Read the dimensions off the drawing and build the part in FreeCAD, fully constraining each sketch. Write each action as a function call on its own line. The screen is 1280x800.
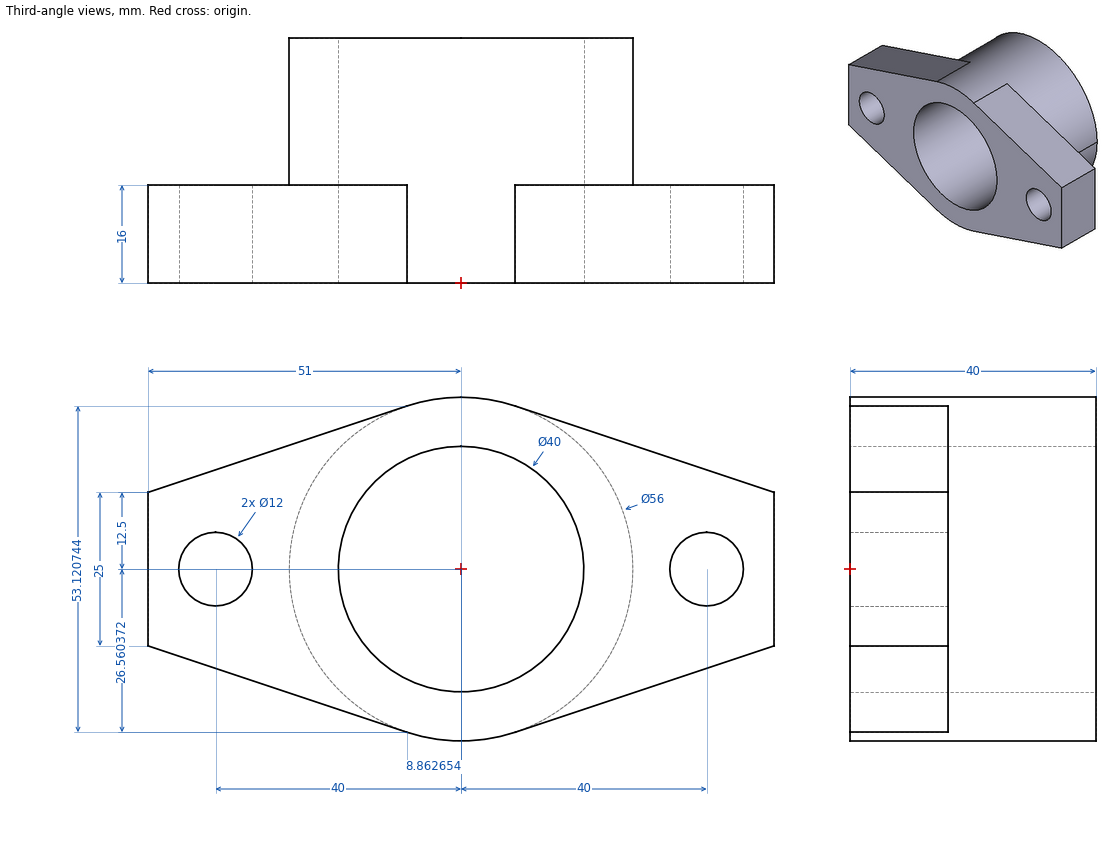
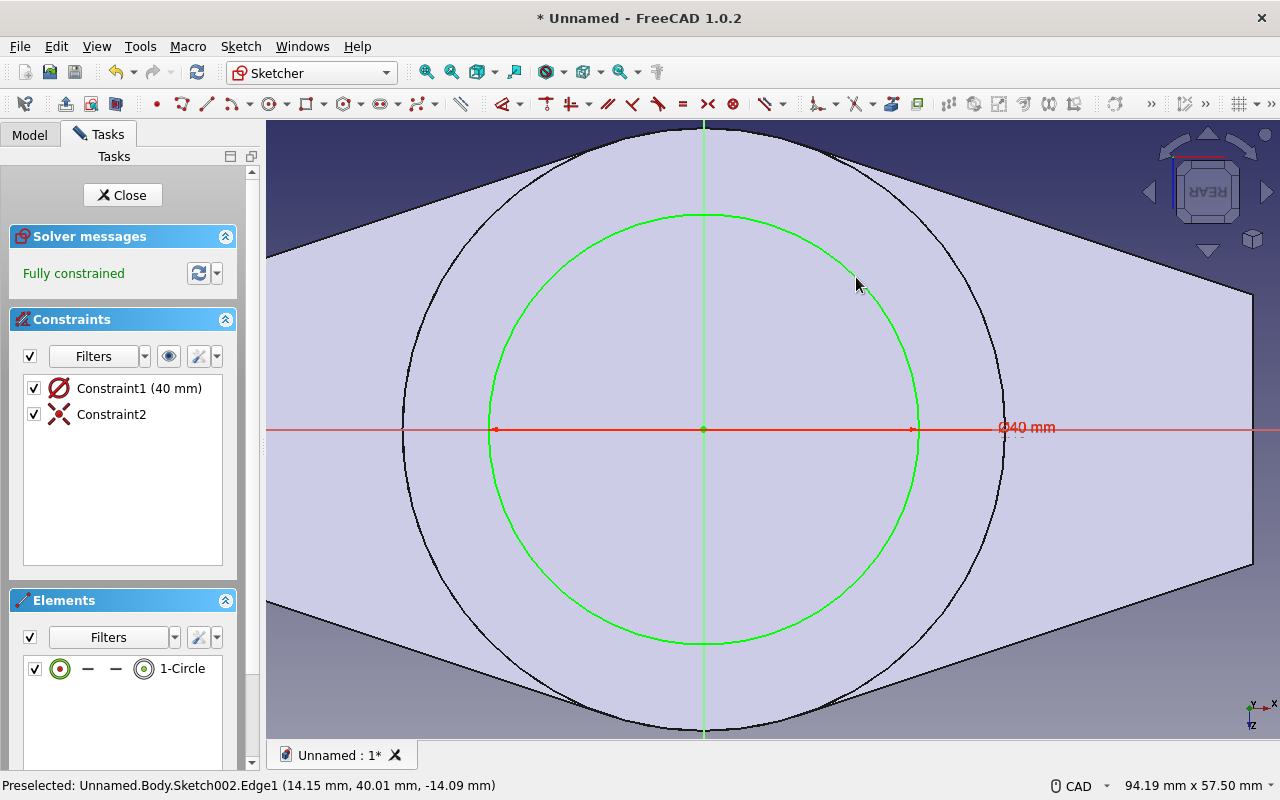
click(123, 195)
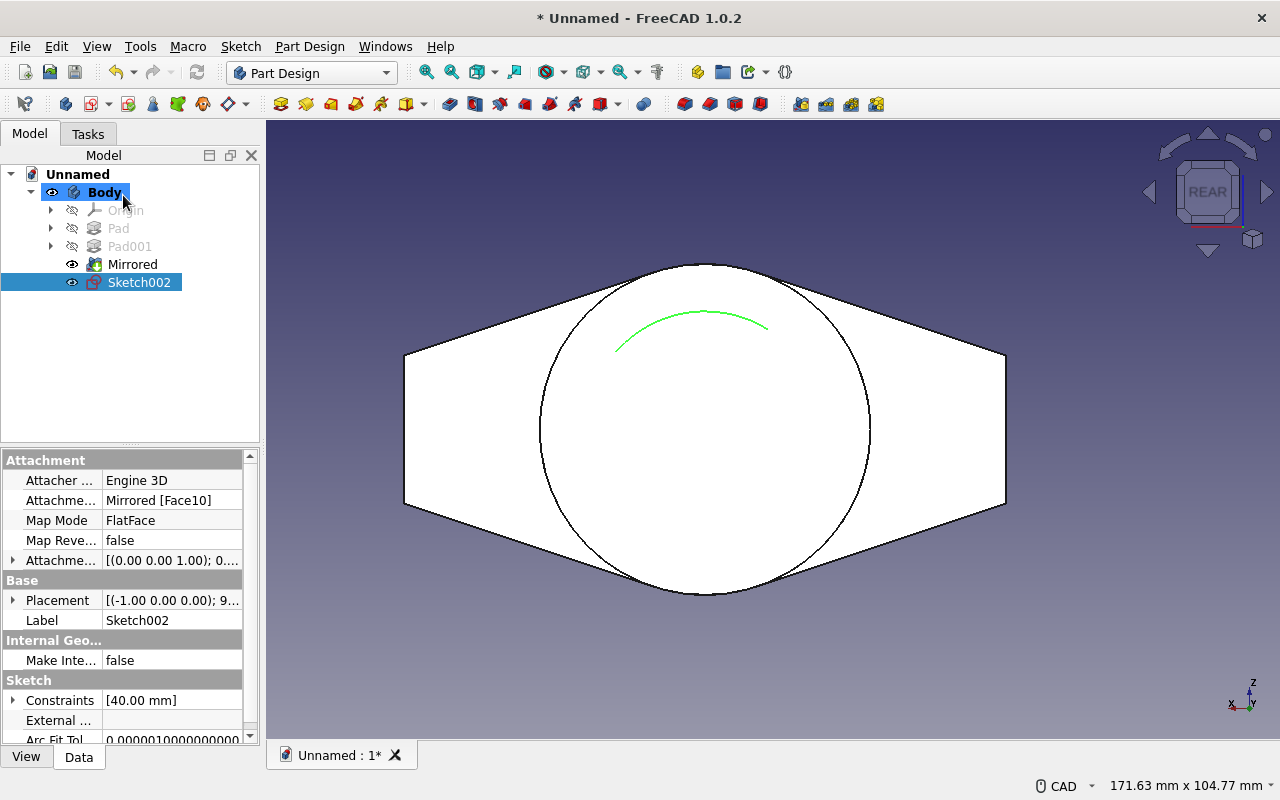
click(450, 104)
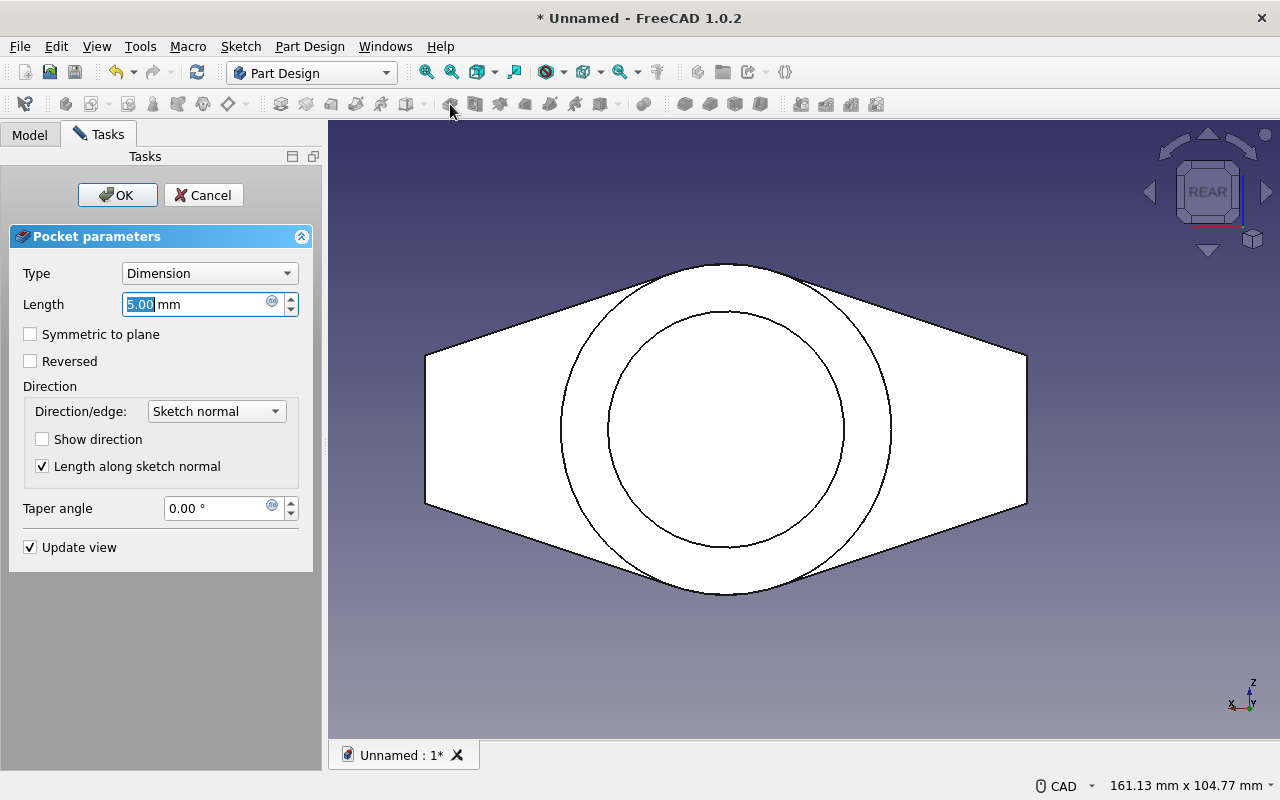
click(210, 274)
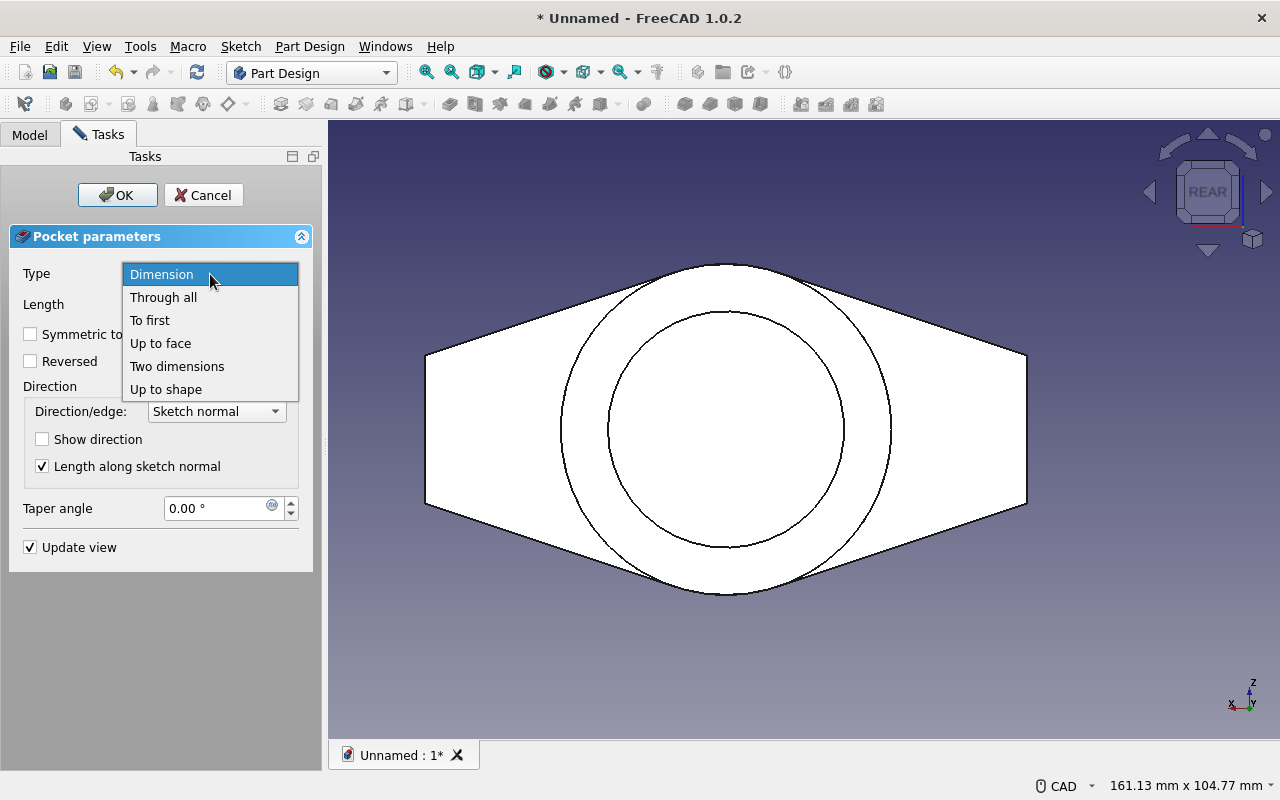
click(208, 298)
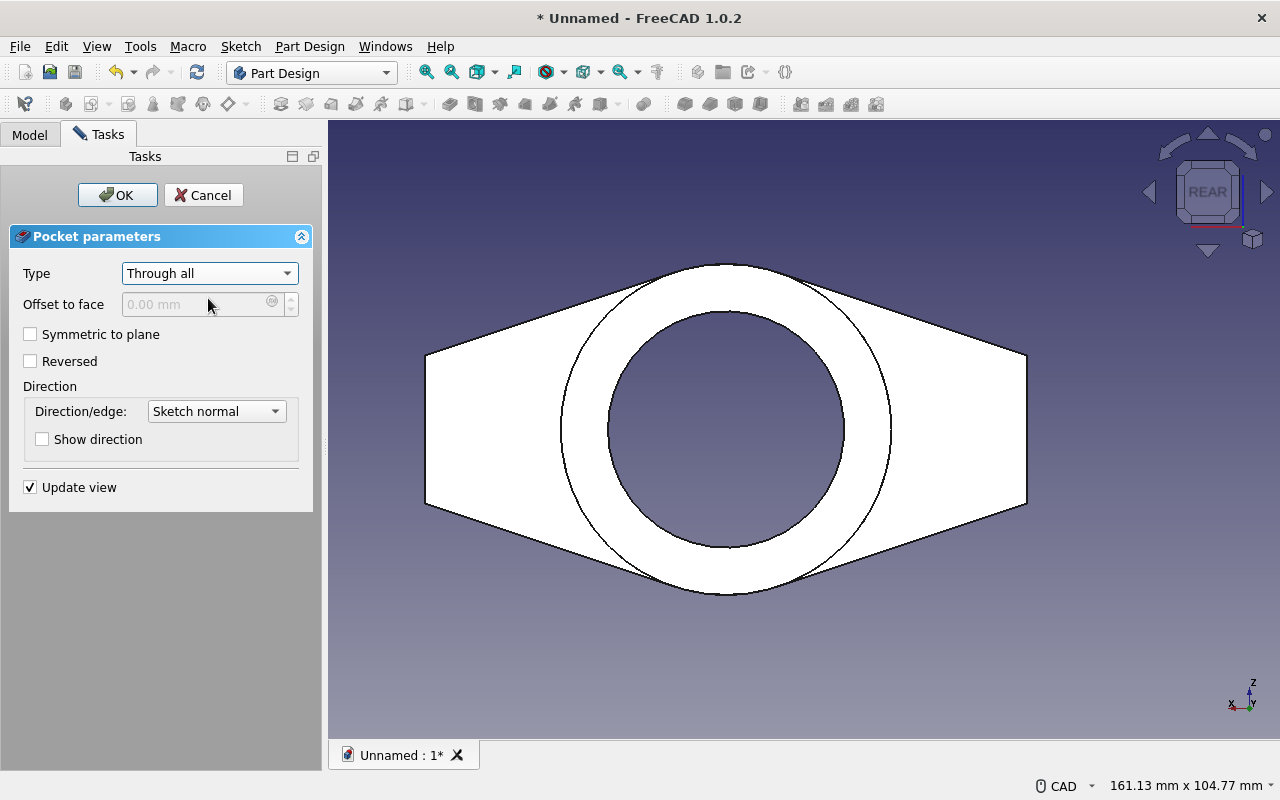
click(118, 195)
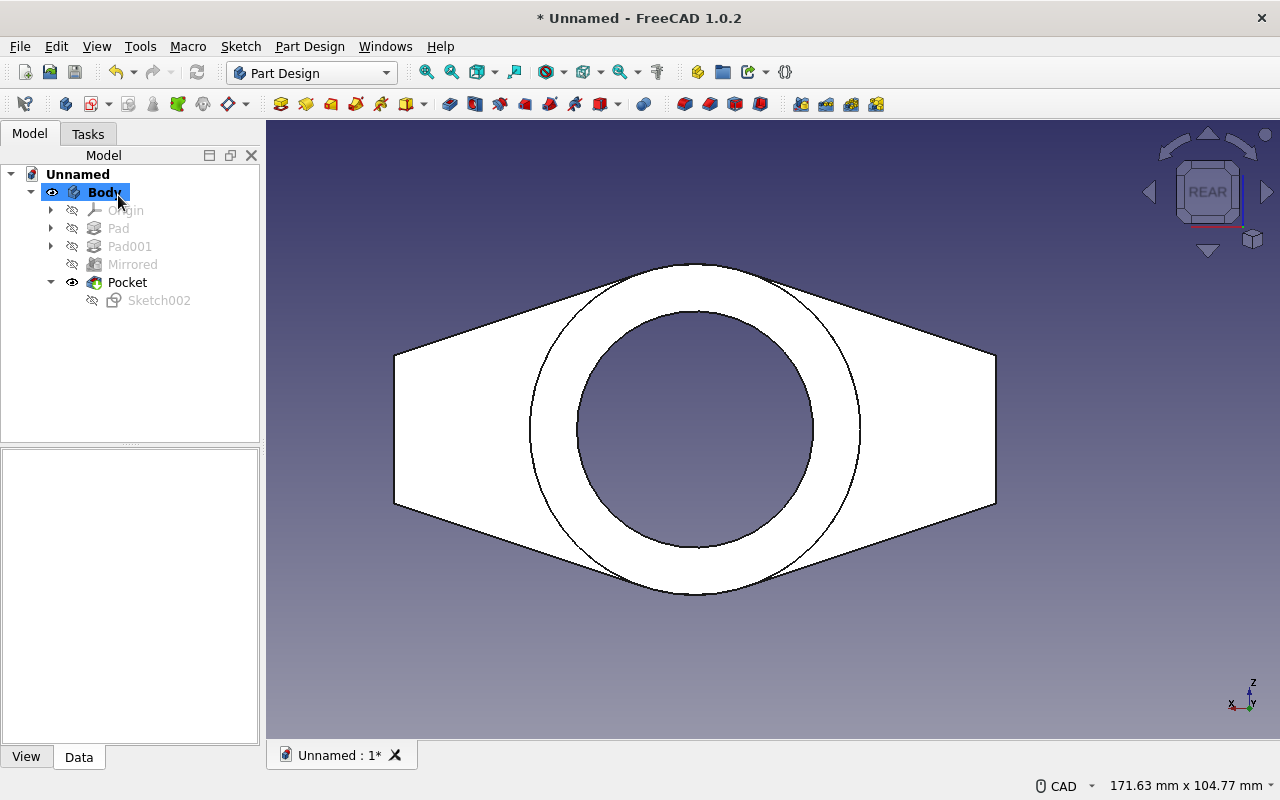
click(447, 429)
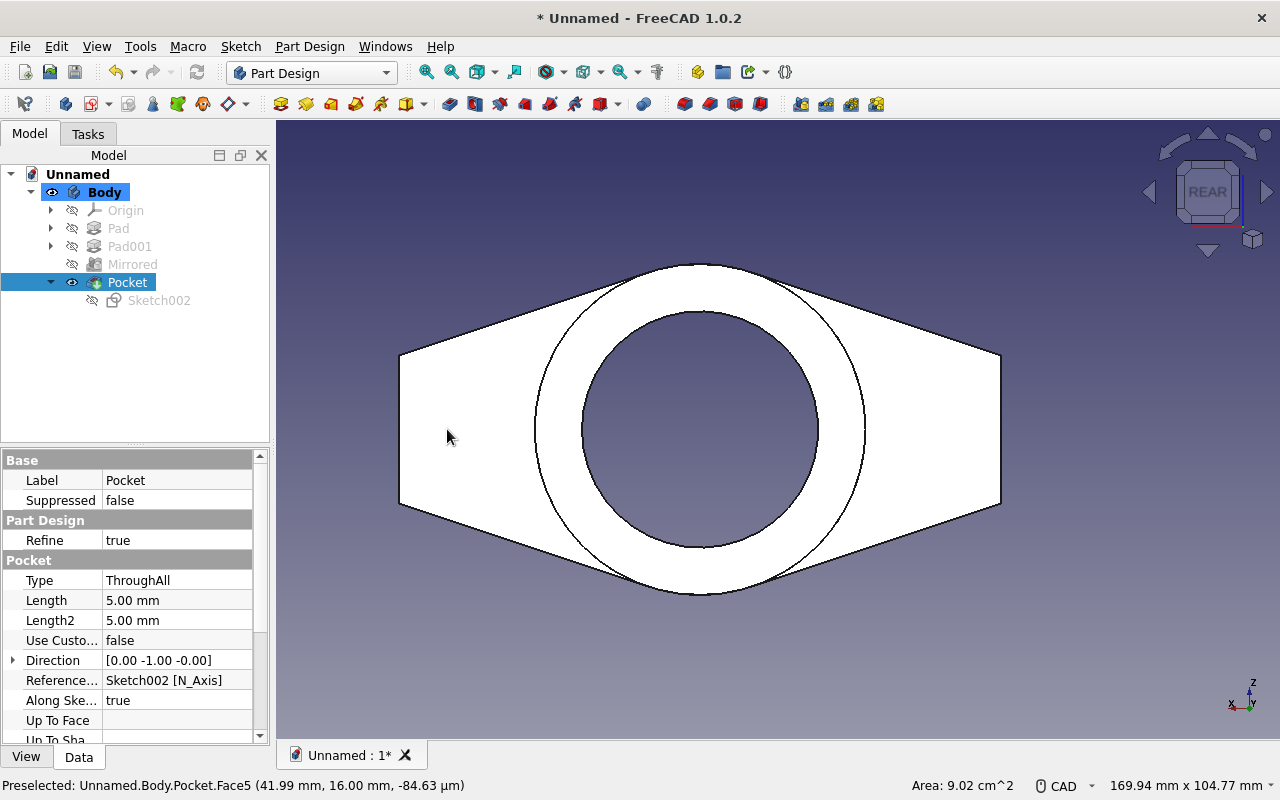
click(90, 104)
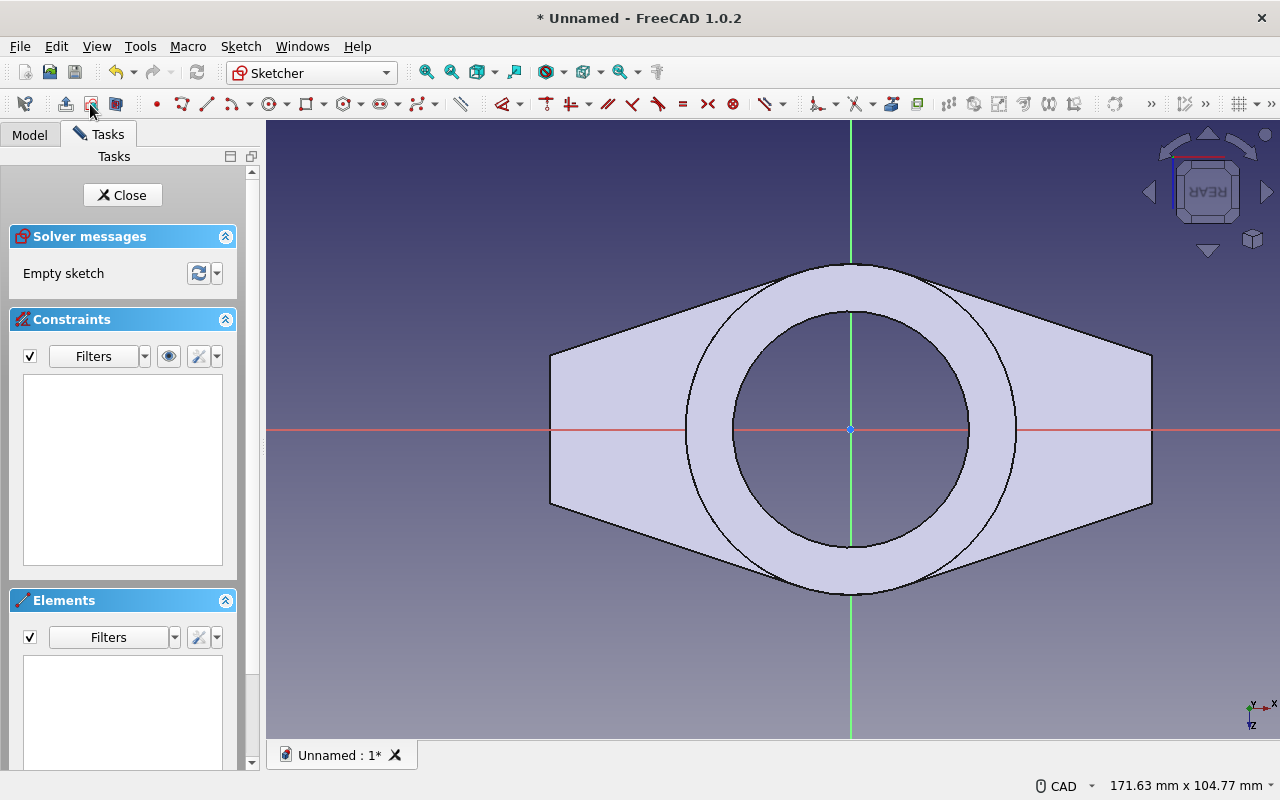
click(116, 104)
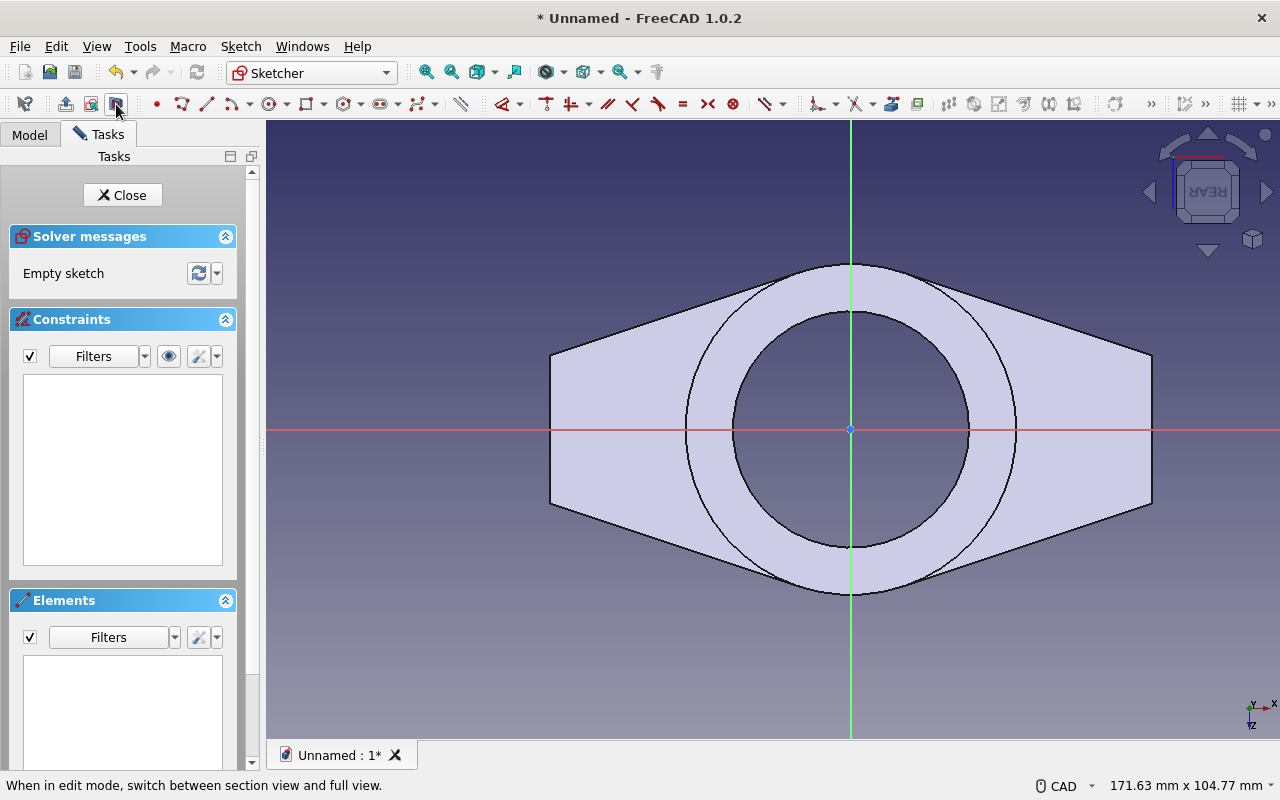
scroll(294, 430, down, 1)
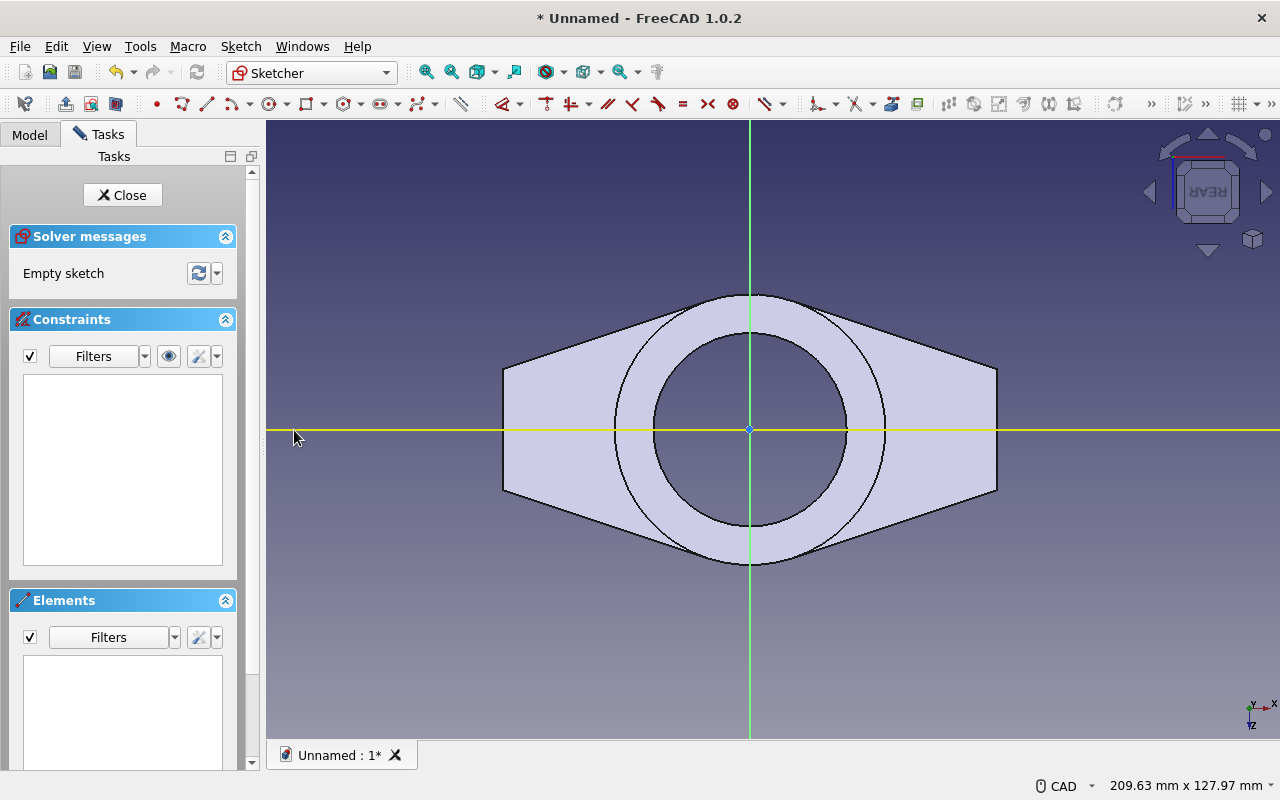
click(268, 104)